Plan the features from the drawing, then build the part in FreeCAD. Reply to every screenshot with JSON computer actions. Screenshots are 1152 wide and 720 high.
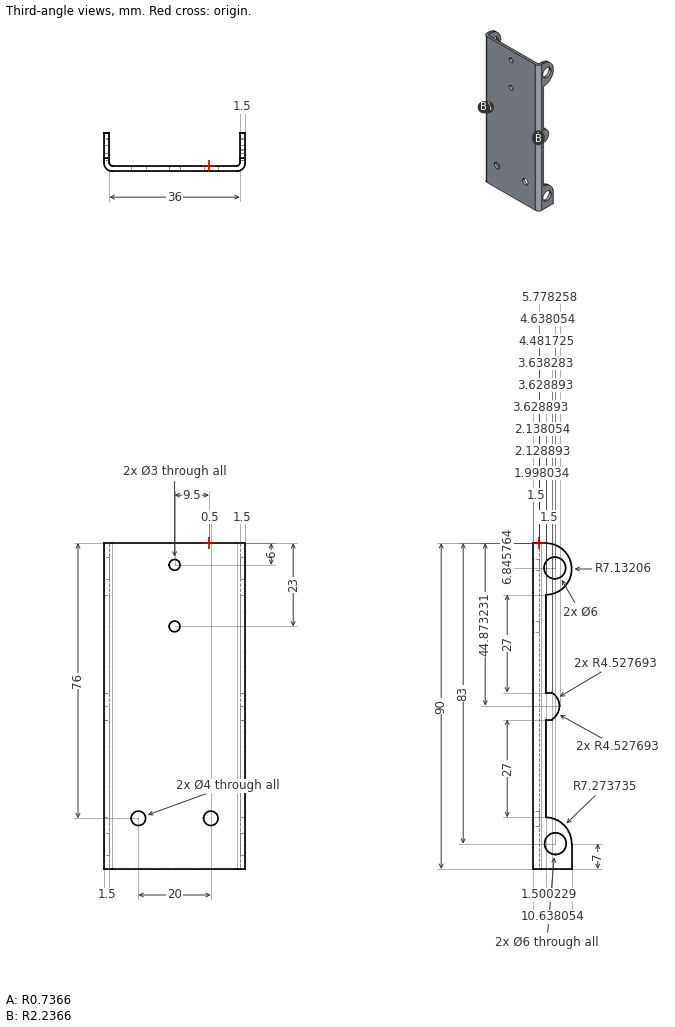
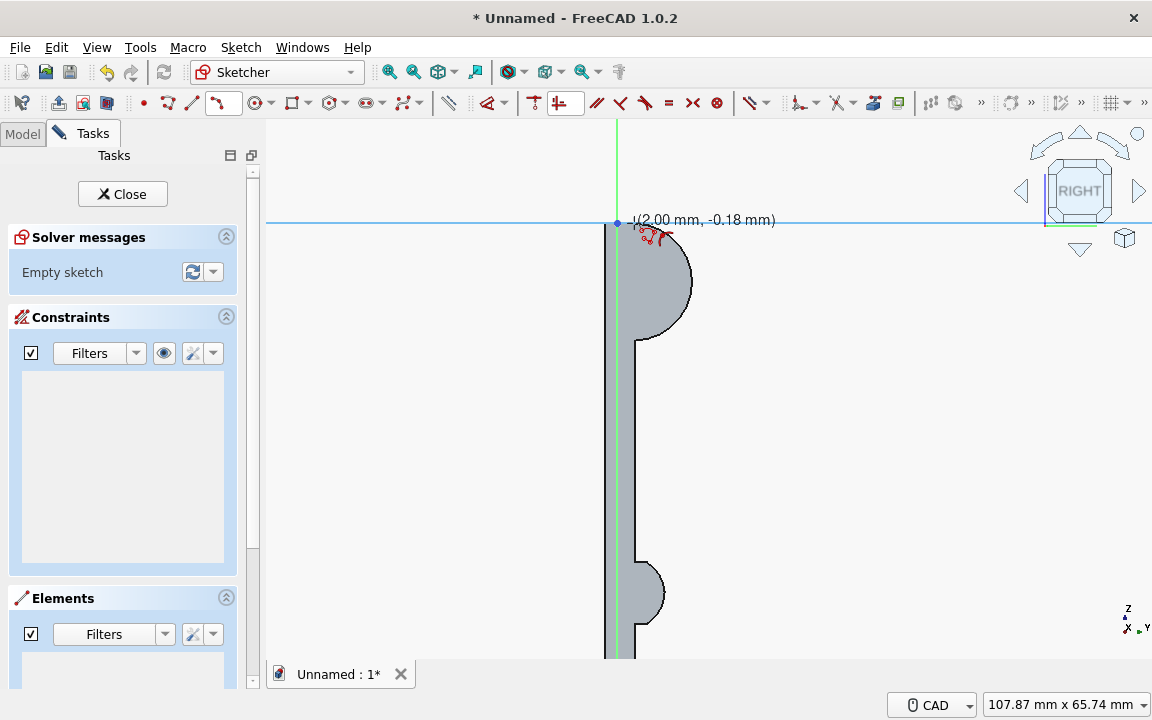
{"action": "left_click", "coordinate": [635, 223]}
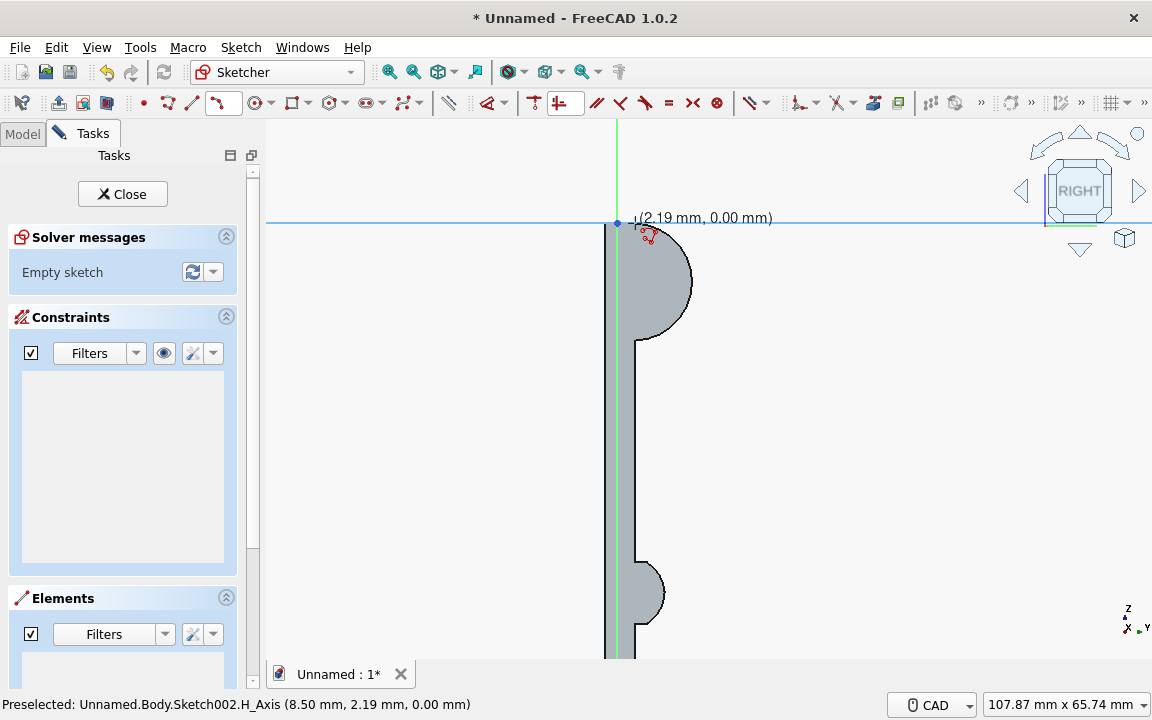
{"action": "scroll", "coordinate": [605, 223], "scroll_direction": "up", "scroll_amount": 2}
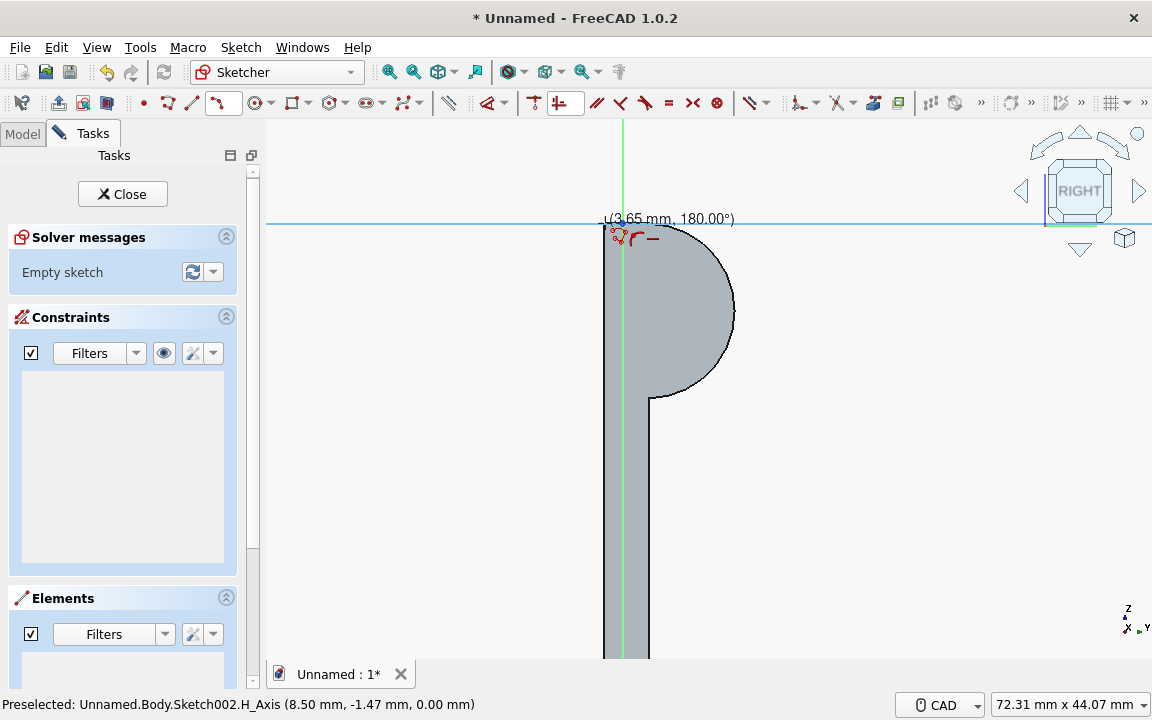
{"action": "left_click", "coordinate": [604, 233]}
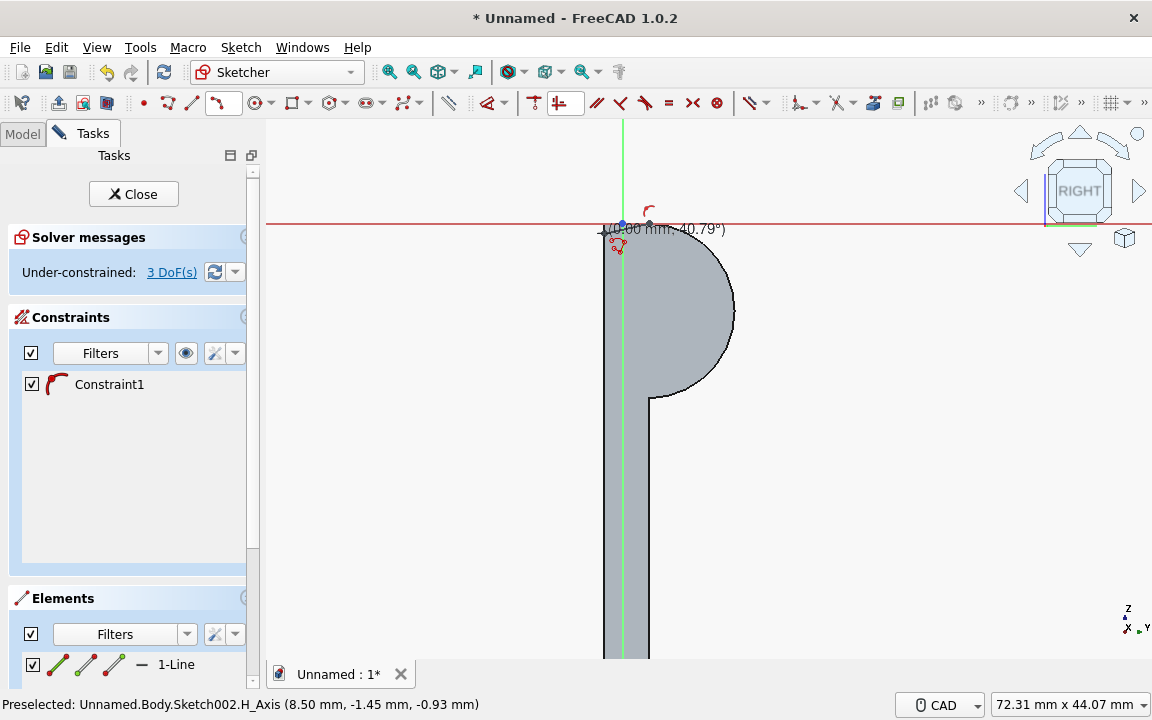
{"action": "scroll", "coordinate": [628, 223], "scroll_direction": "down", "scroll_amount": 6}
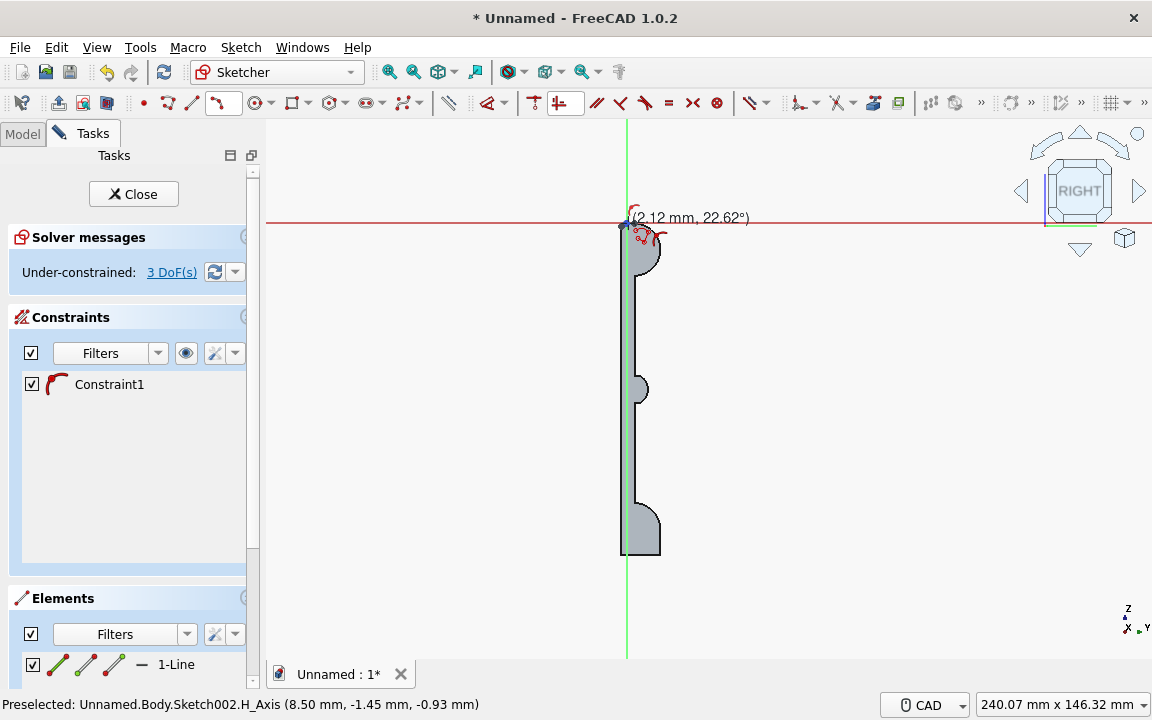
{"action": "scroll", "coordinate": [621, 555], "scroll_direction": "up", "scroll_amount": 6}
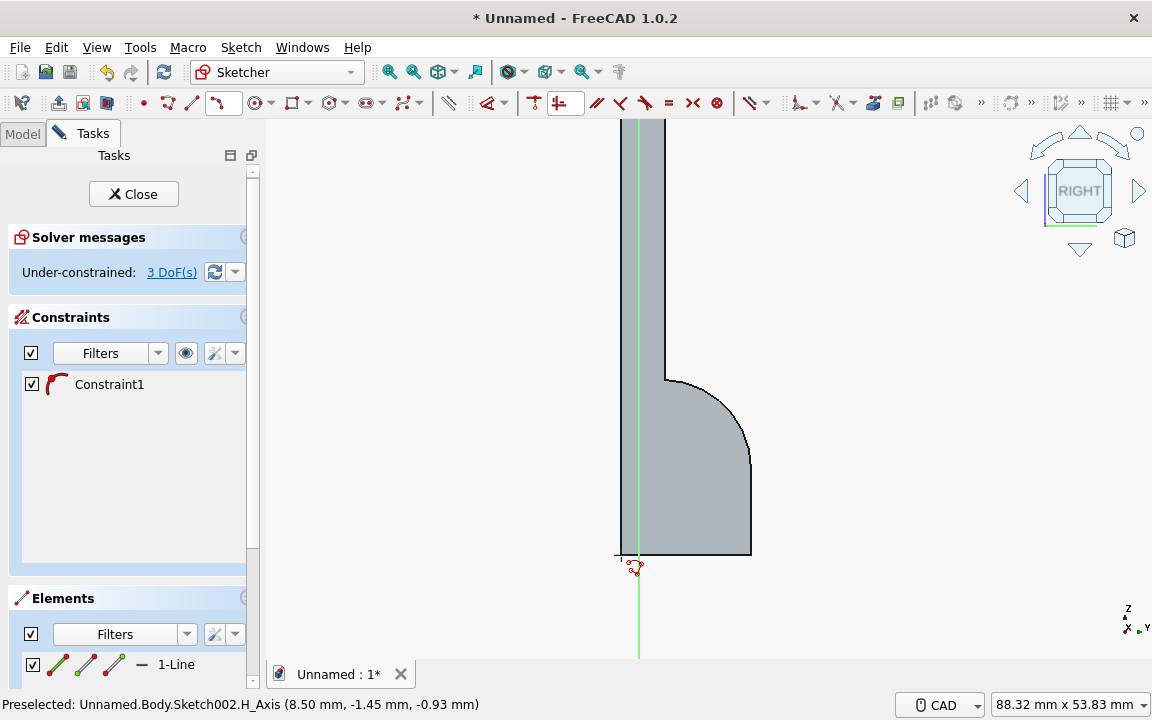
{"action": "left_click", "coordinate": [620, 555]}
{"action": "left_click", "coordinate": [751, 555]}
{"action": "left_click", "coordinate": [751, 469]}
{"action": "right_click", "coordinate": [751, 469]}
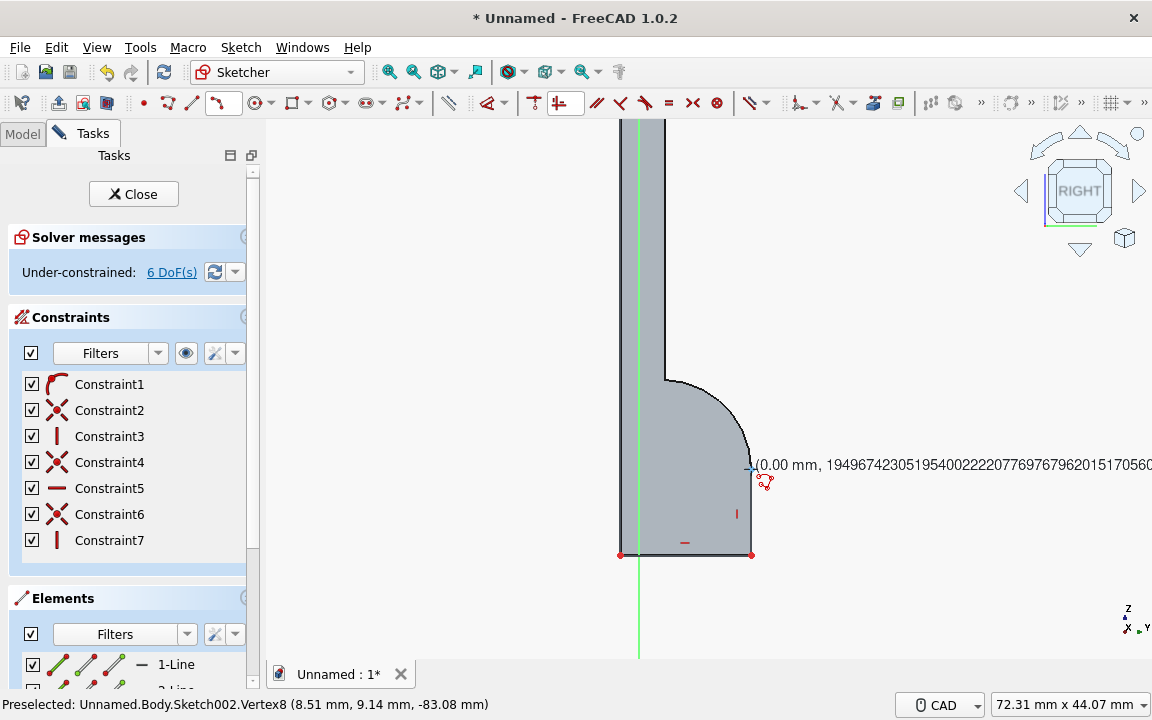
{"action": "left_click", "coordinate": [665, 380]}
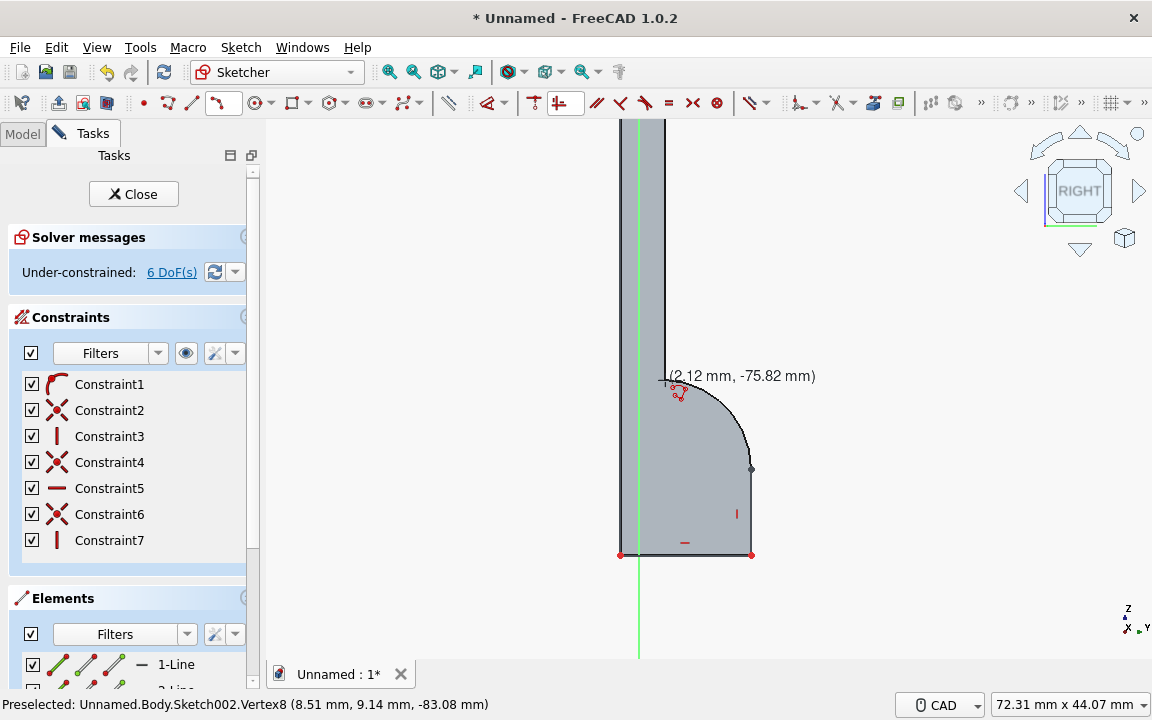
{"action": "scroll", "coordinate": [621, 555], "scroll_direction": "down", "scroll_amount": 6}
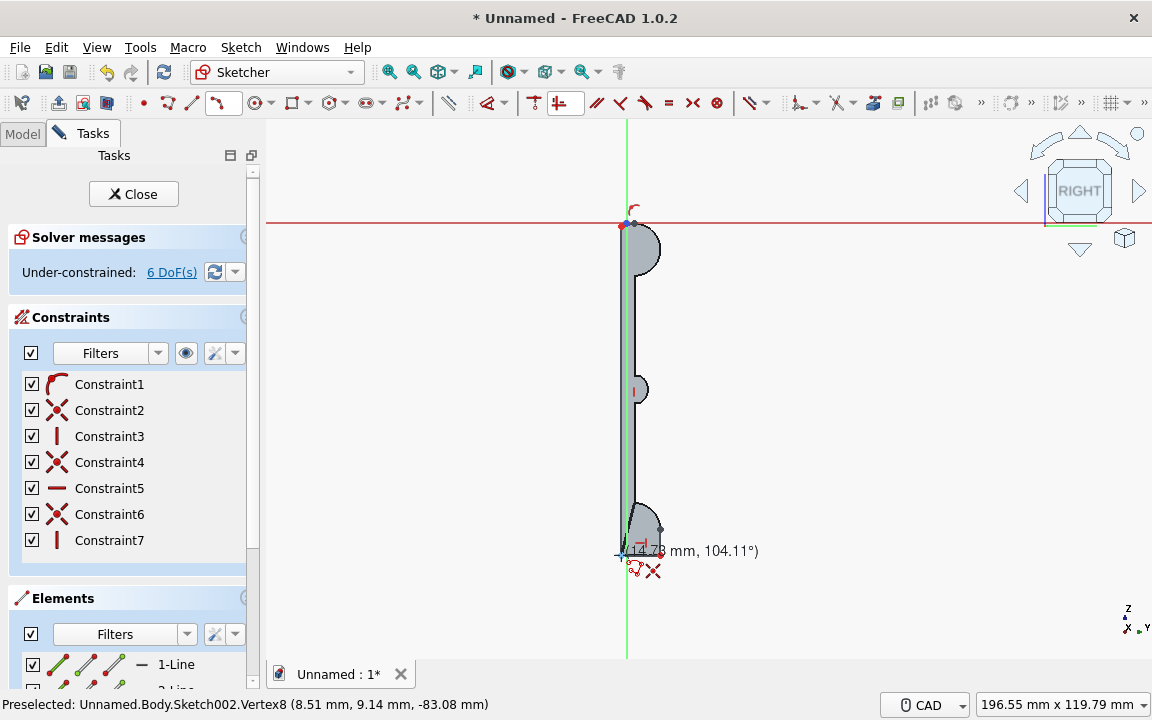
{"action": "scroll", "coordinate": [635, 403], "scroll_direction": "up", "scroll_amount": 4}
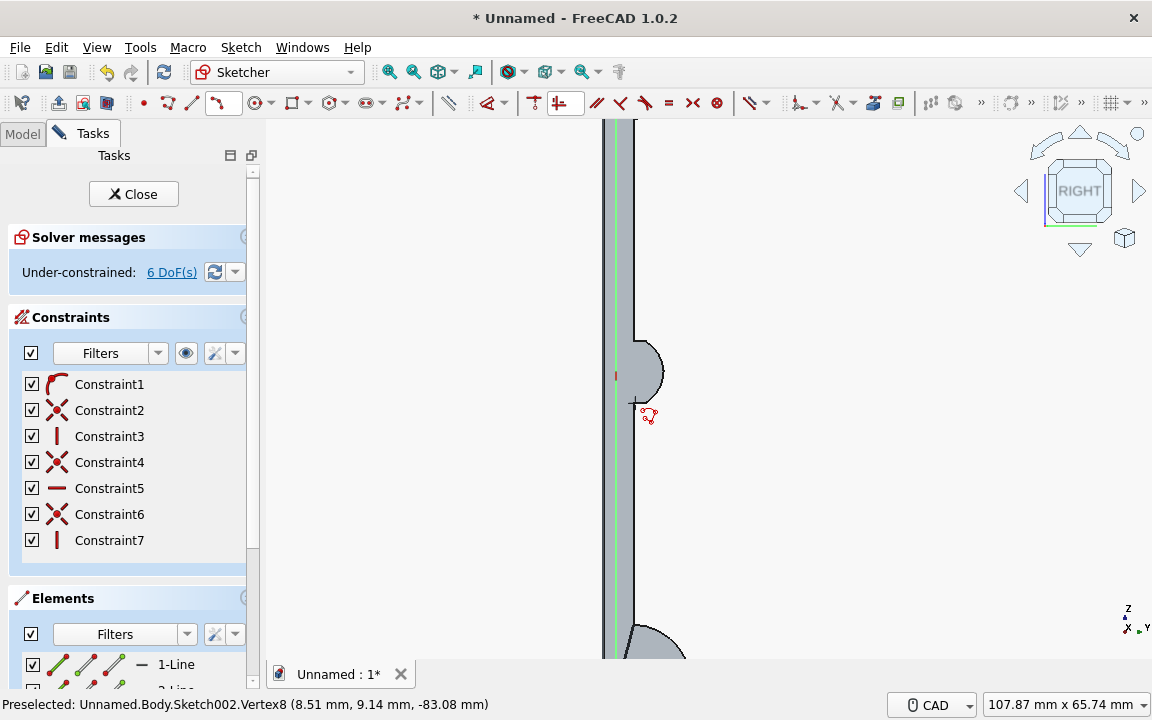
{"action": "left_click", "coordinate": [633, 403]}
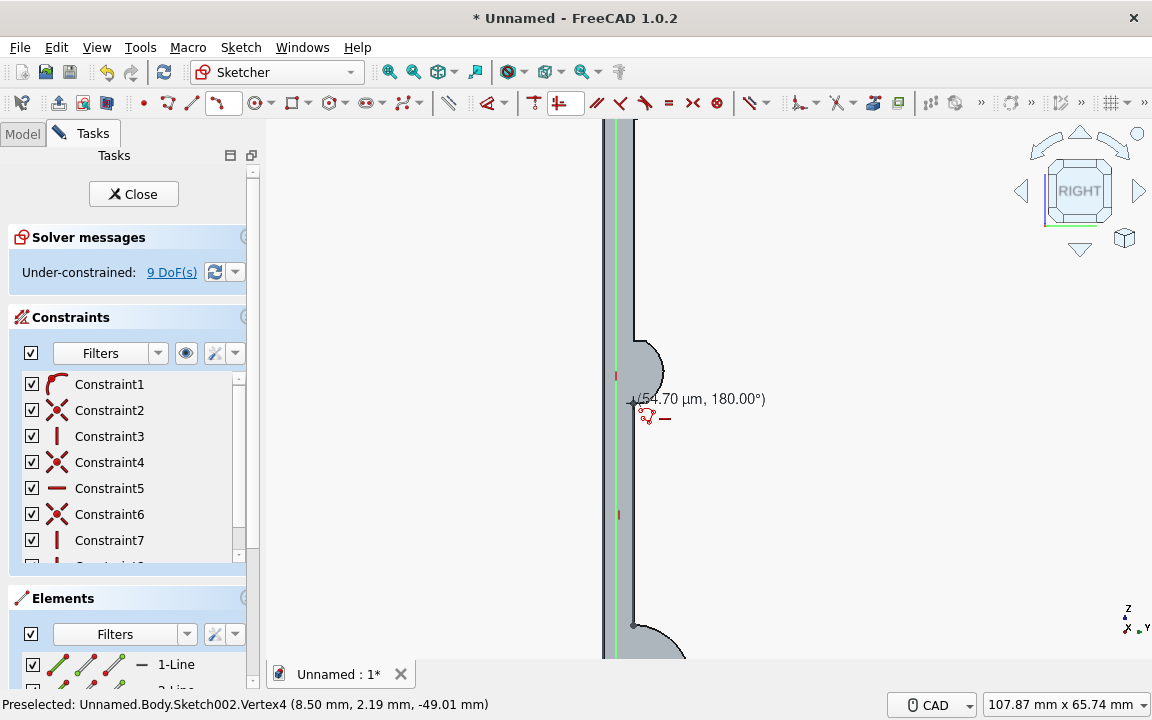
{"action": "scroll", "coordinate": [646, 403], "scroll_direction": "up", "scroll_amount": 2}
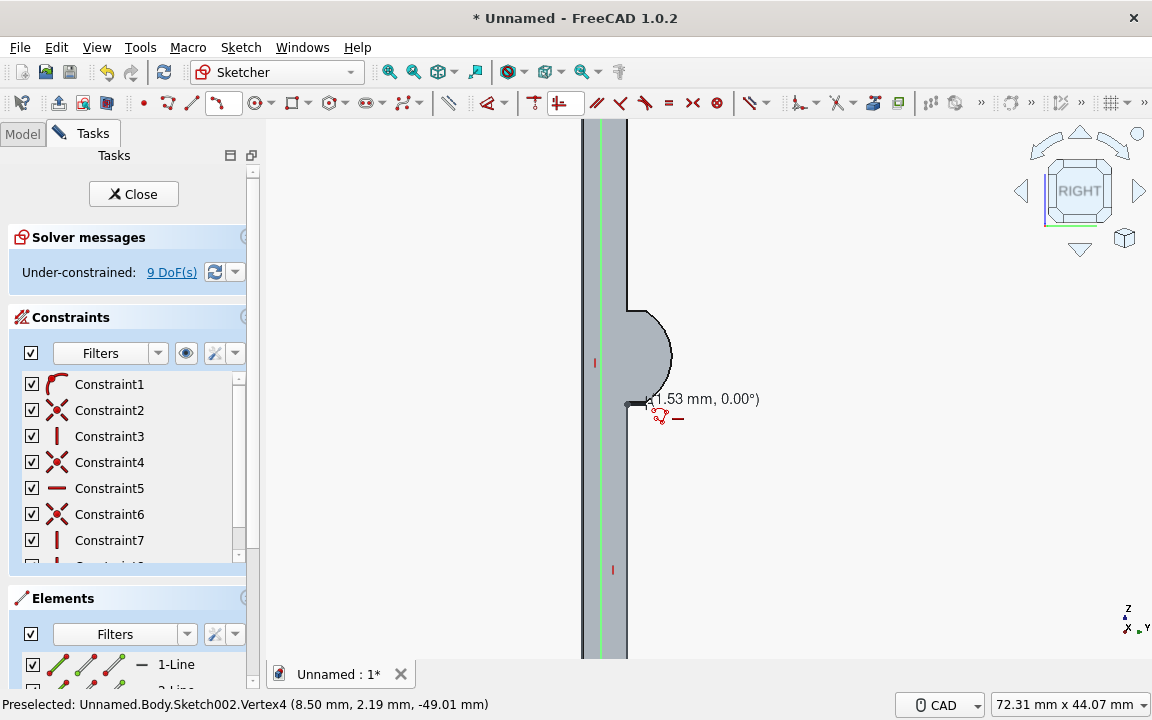
{"action": "left_click", "coordinate": [646, 403]}
{"action": "right_click", "coordinate": [646, 403]}